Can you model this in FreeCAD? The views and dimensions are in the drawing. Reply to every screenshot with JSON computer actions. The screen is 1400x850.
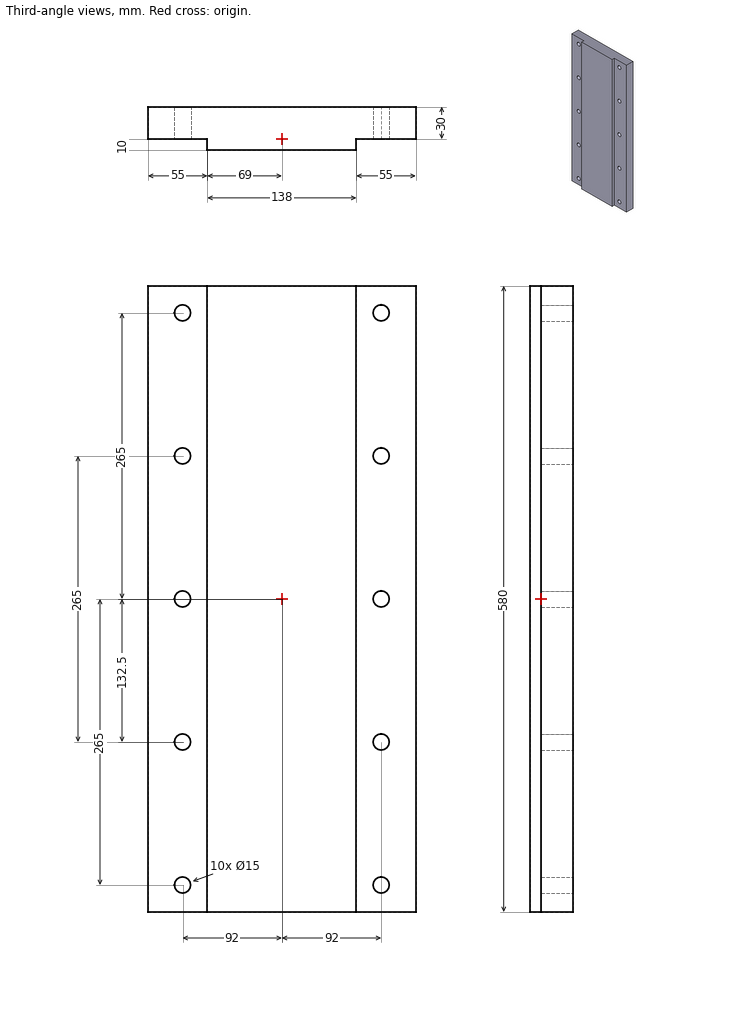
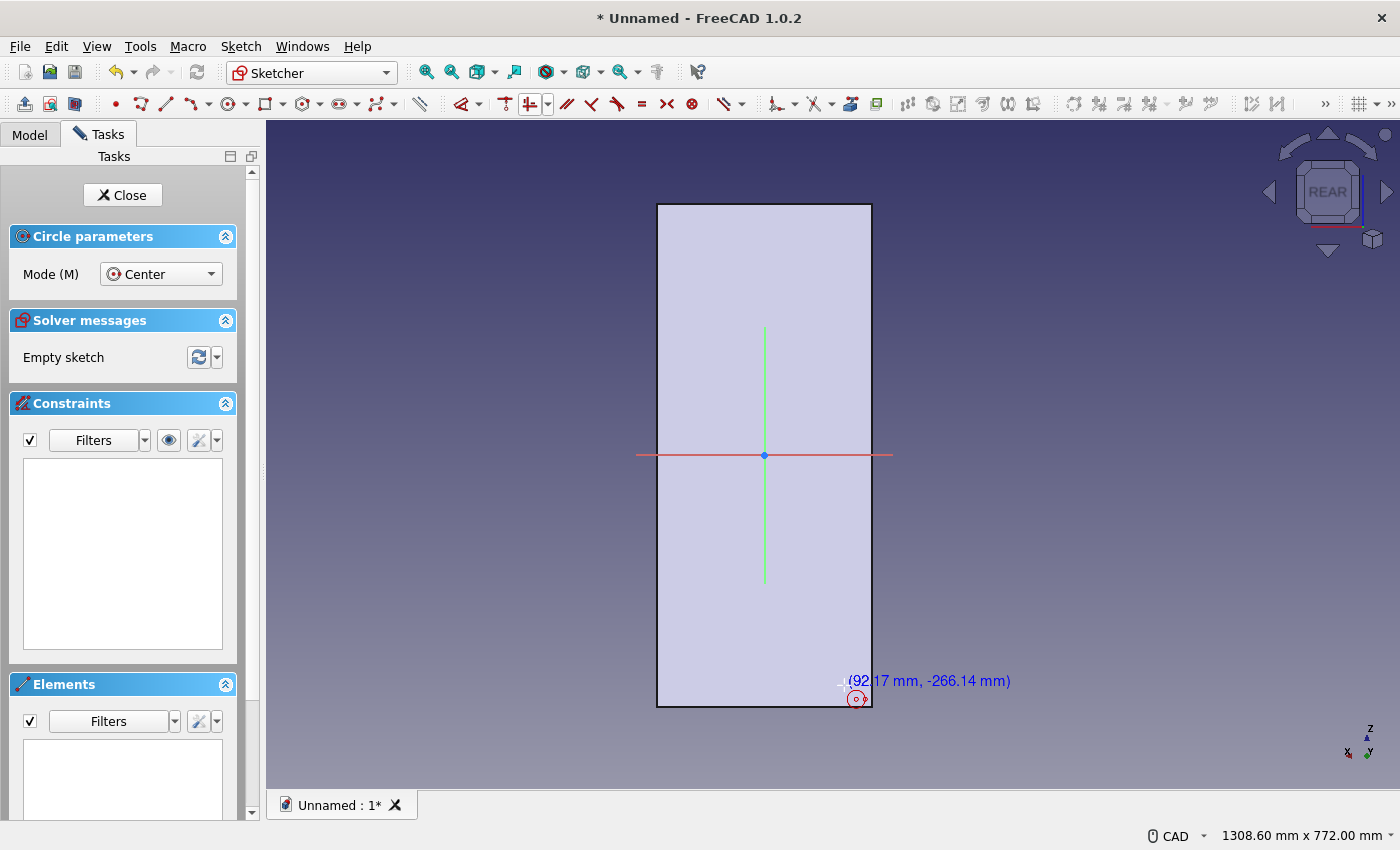
{"action": "left_click", "coordinate": [844, 685]}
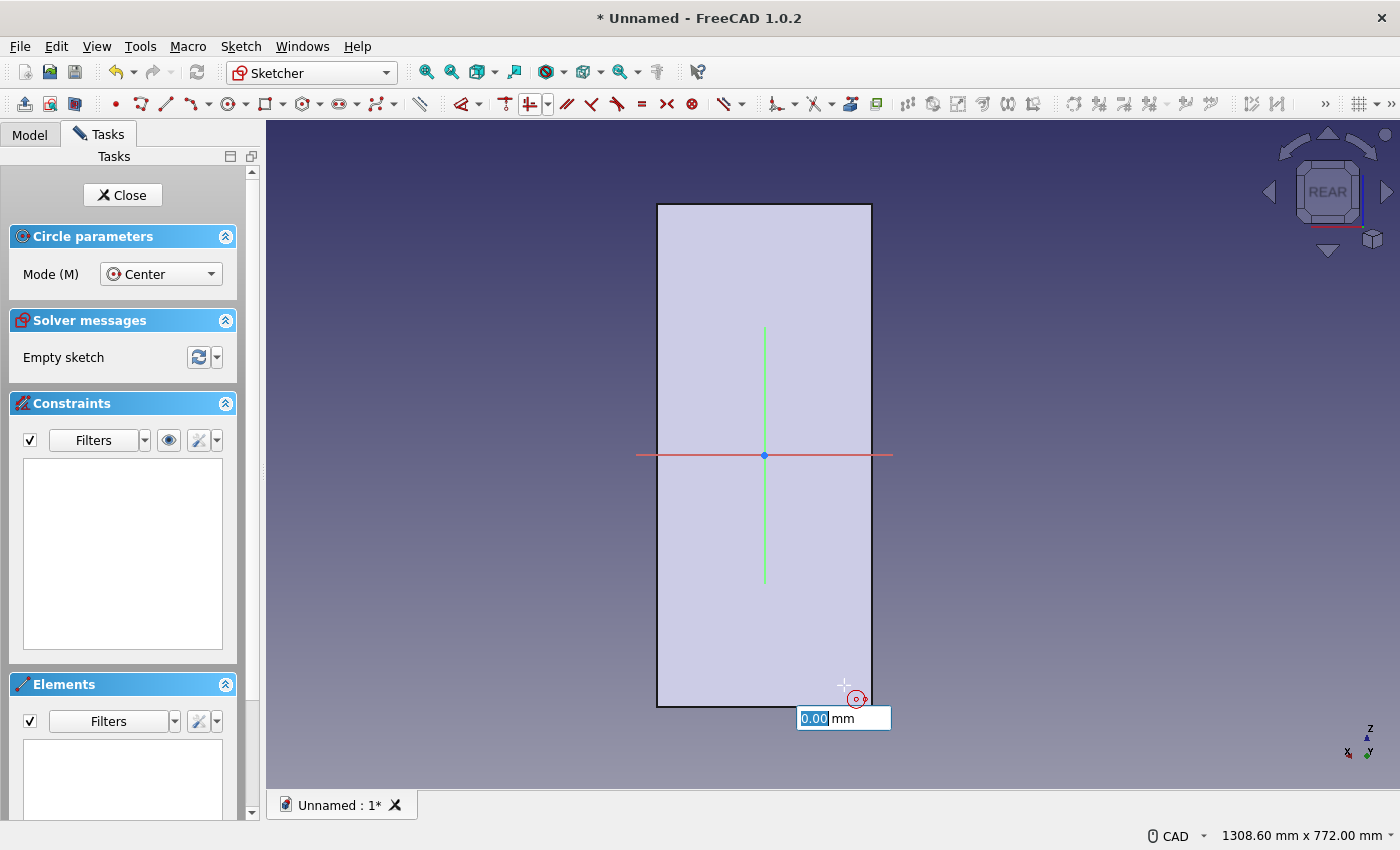
{"action": "scroll", "coordinate": [849, 680], "scroll_direction": "up", "scroll_amount": 5}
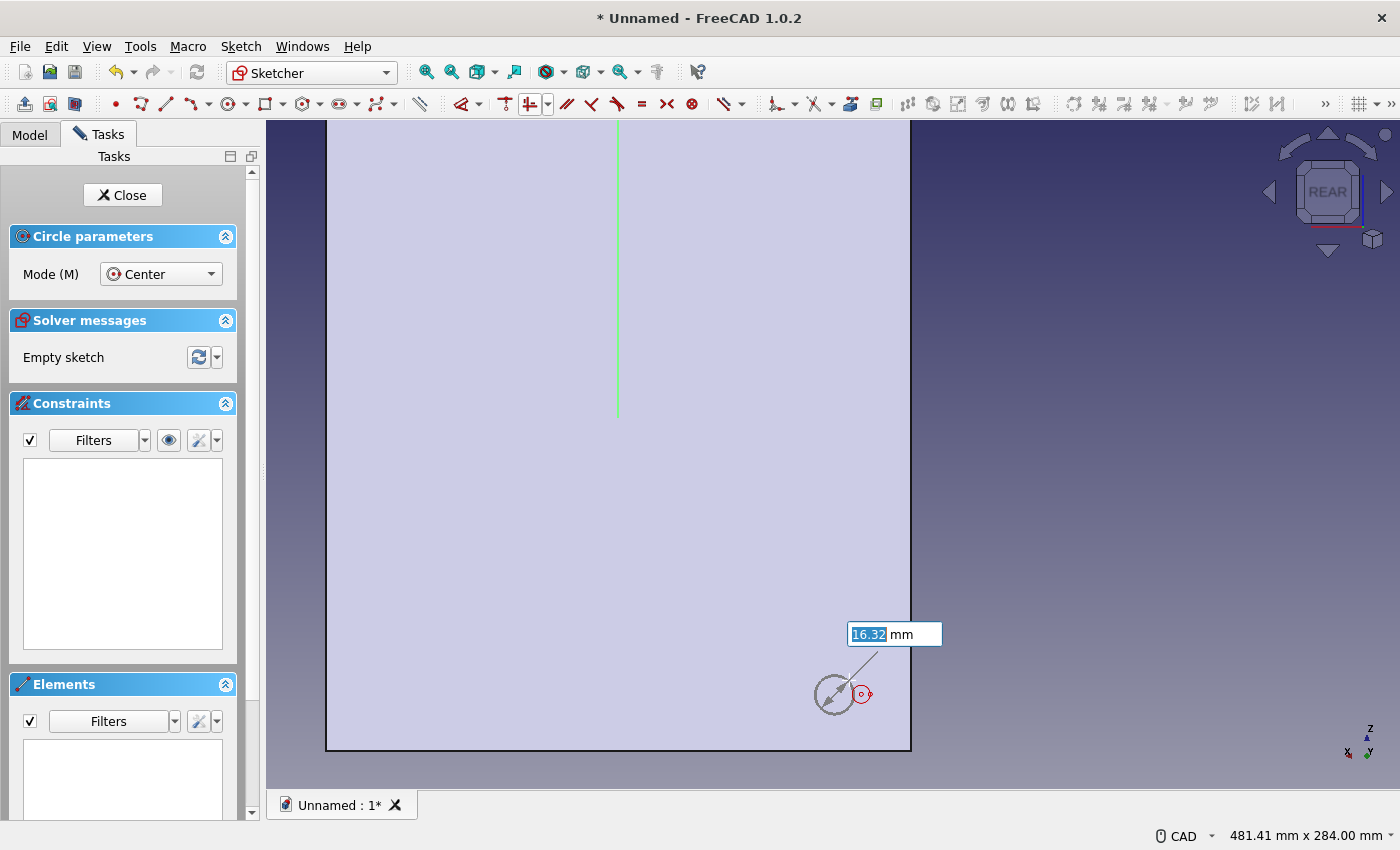
{"action": "left_click", "coordinate": [848, 679]}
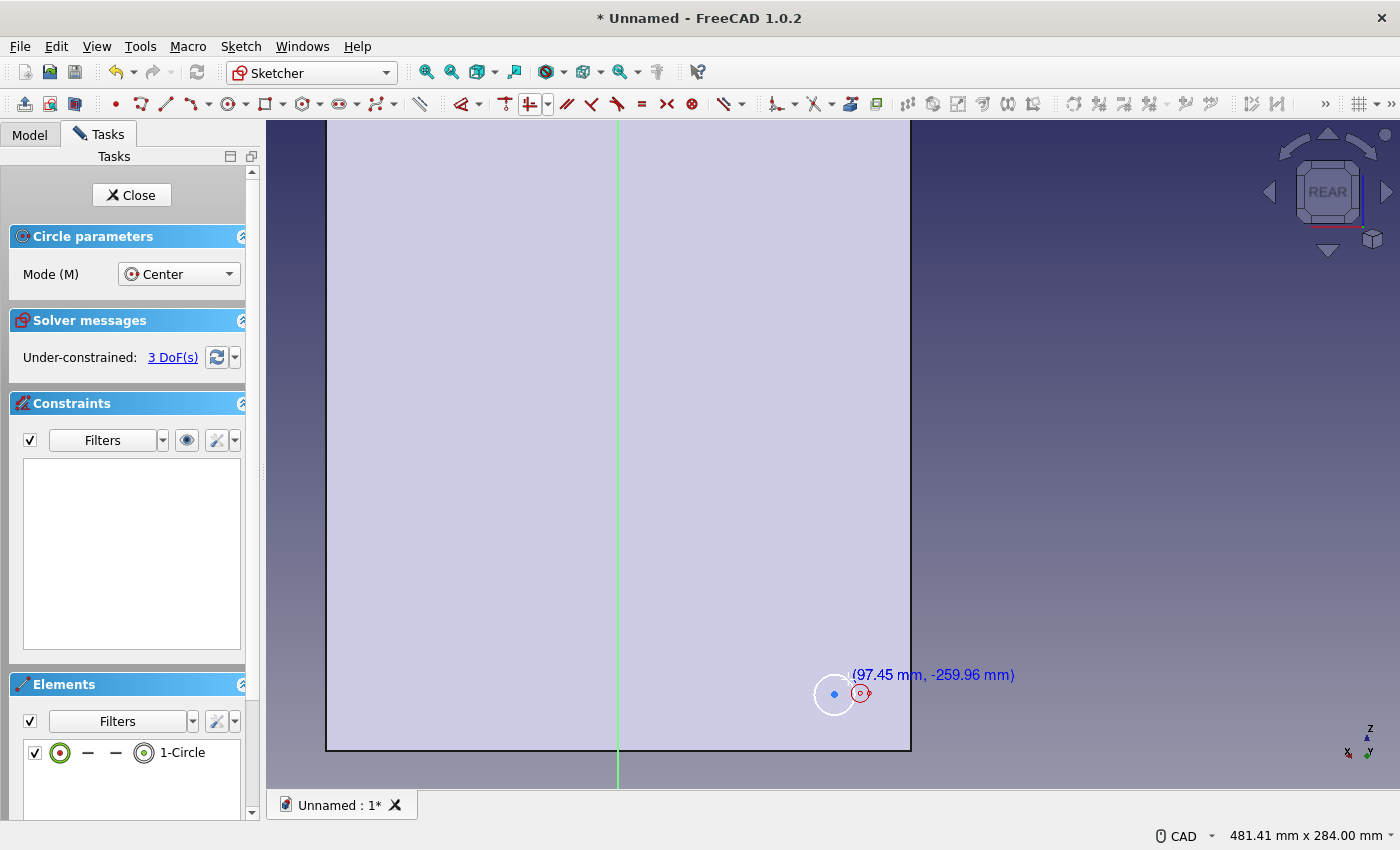
{"action": "scroll", "coordinate": [835, 380], "scroll_direction": "up", "scroll_amount": 2}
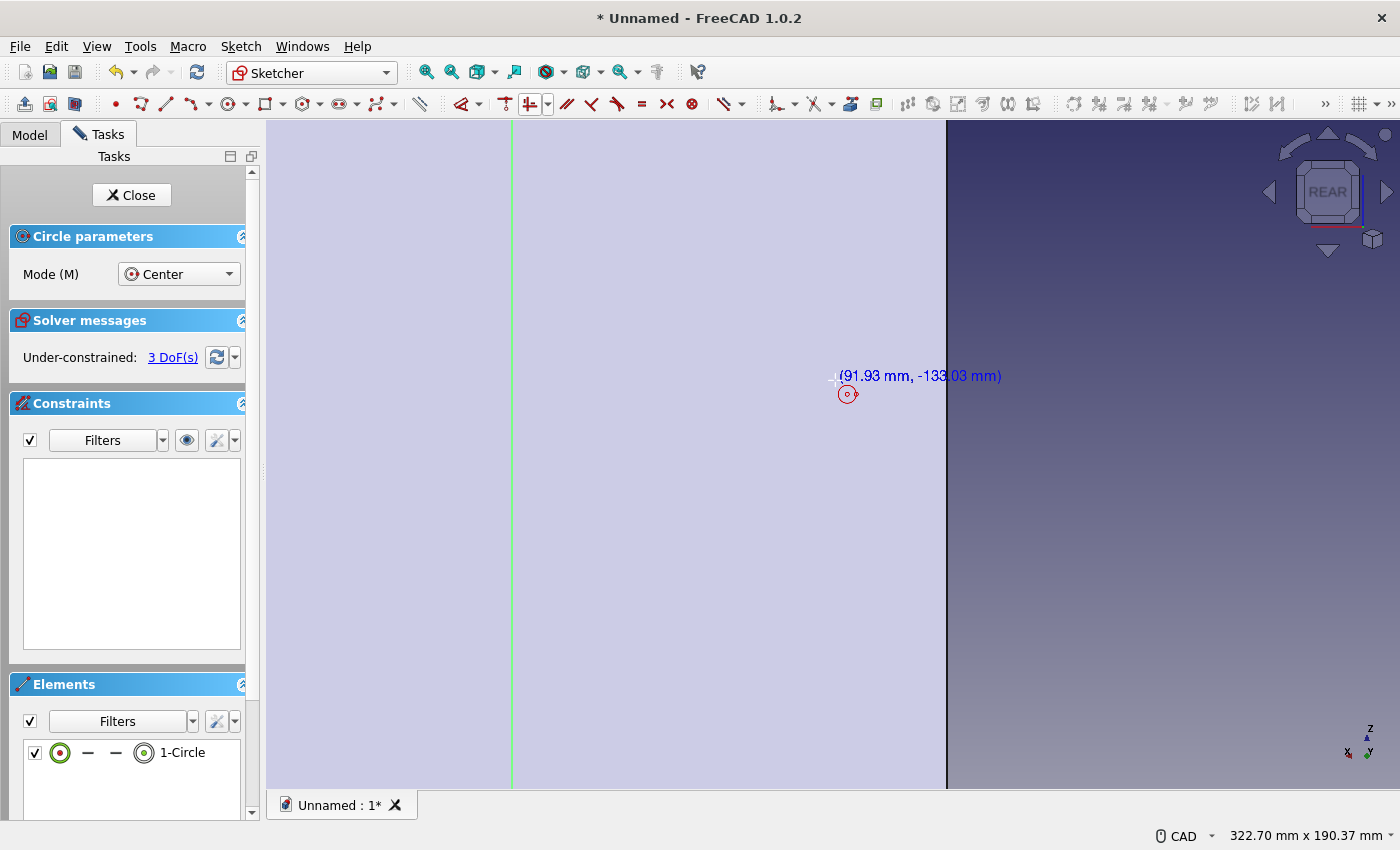
{"action": "scroll", "coordinate": [847, 631], "scroll_direction": "down", "scroll_amount": 7}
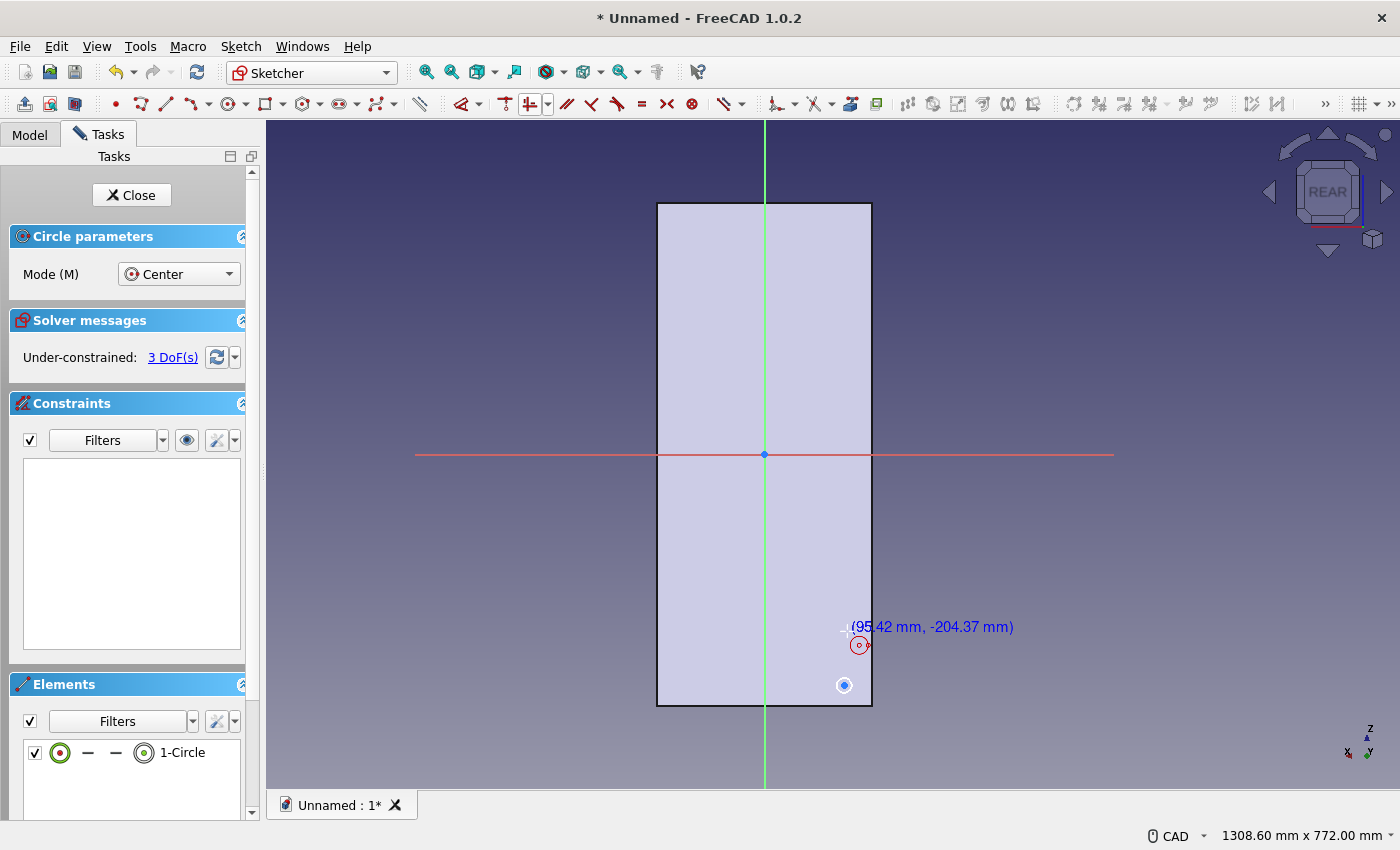
{"action": "left_click", "coordinate": [844, 570]}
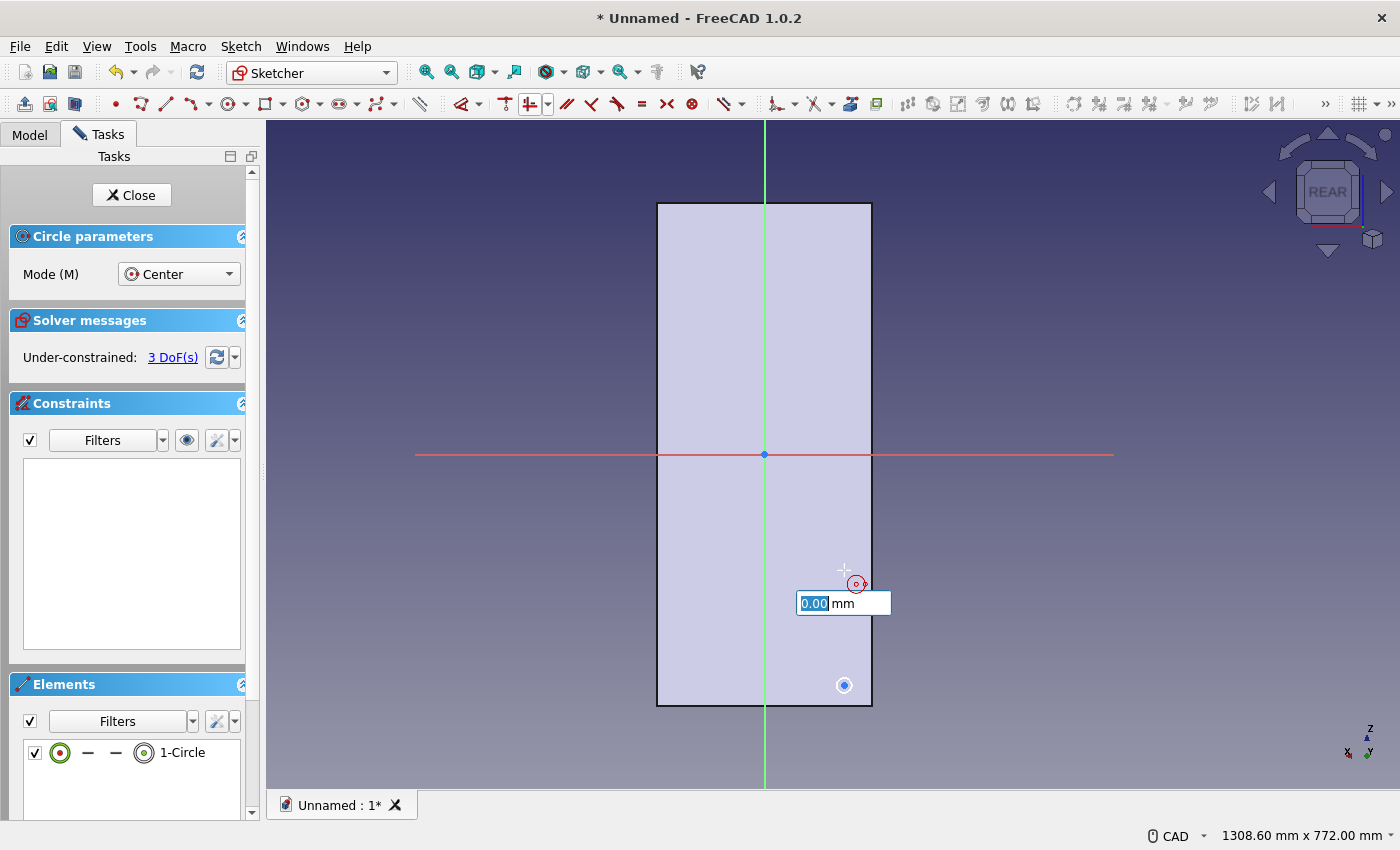
{"action": "scroll", "coordinate": [849, 565], "scroll_direction": "up", "scroll_amount": 5}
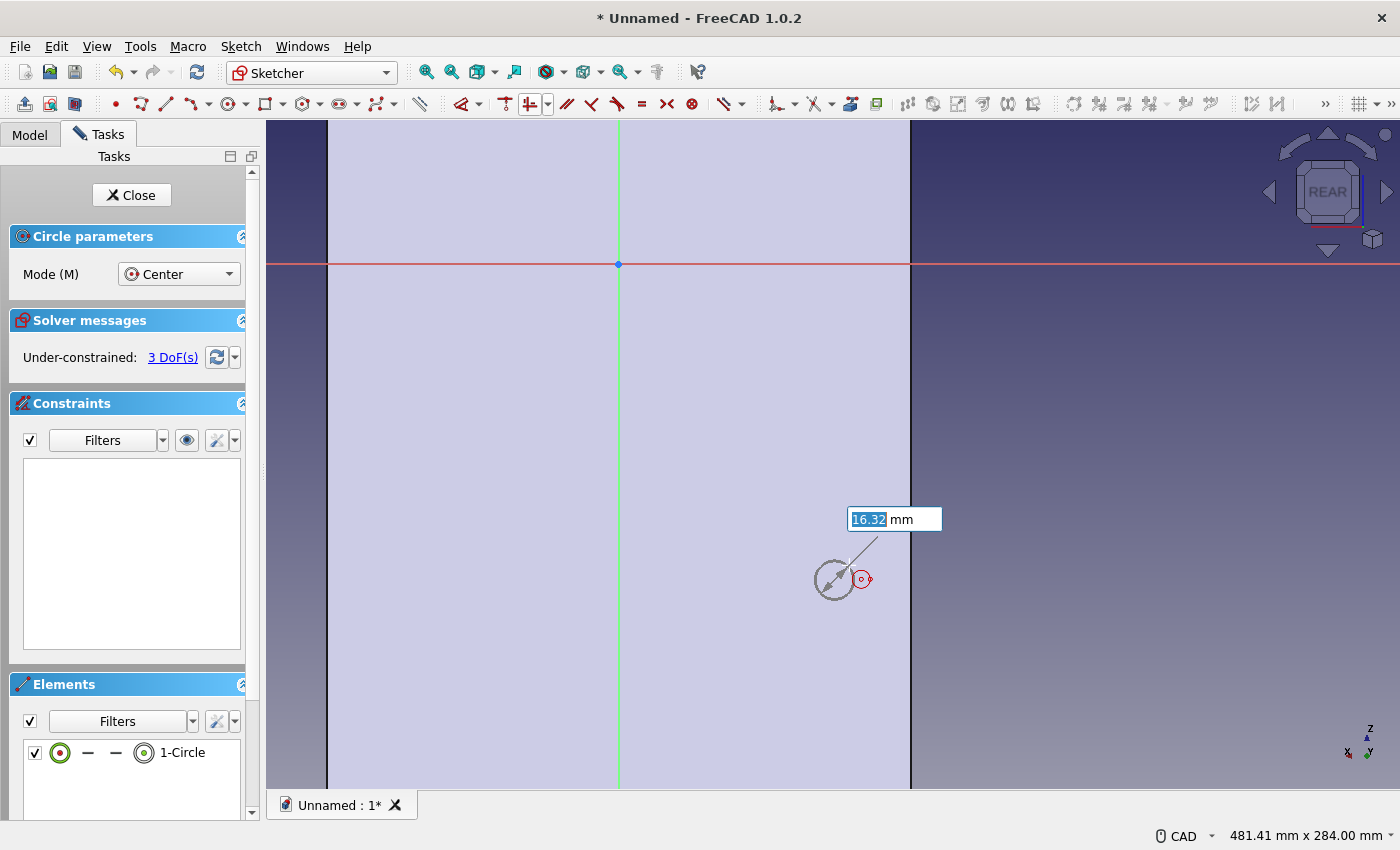
{"action": "left_click", "coordinate": [848, 564]}